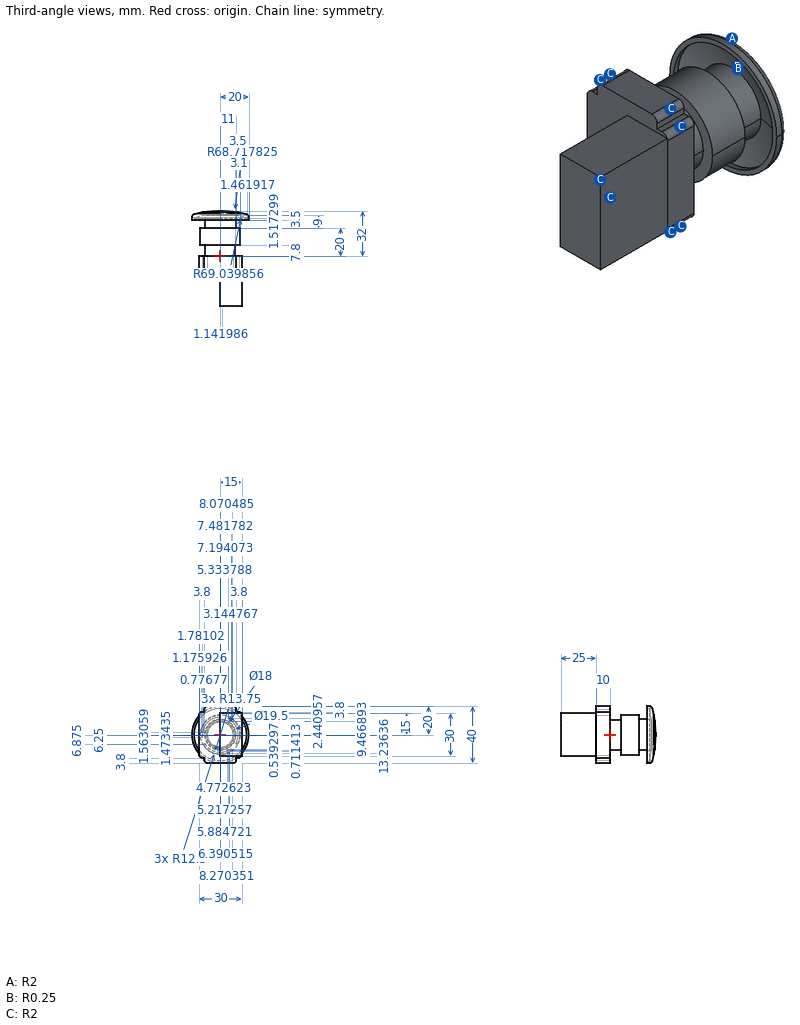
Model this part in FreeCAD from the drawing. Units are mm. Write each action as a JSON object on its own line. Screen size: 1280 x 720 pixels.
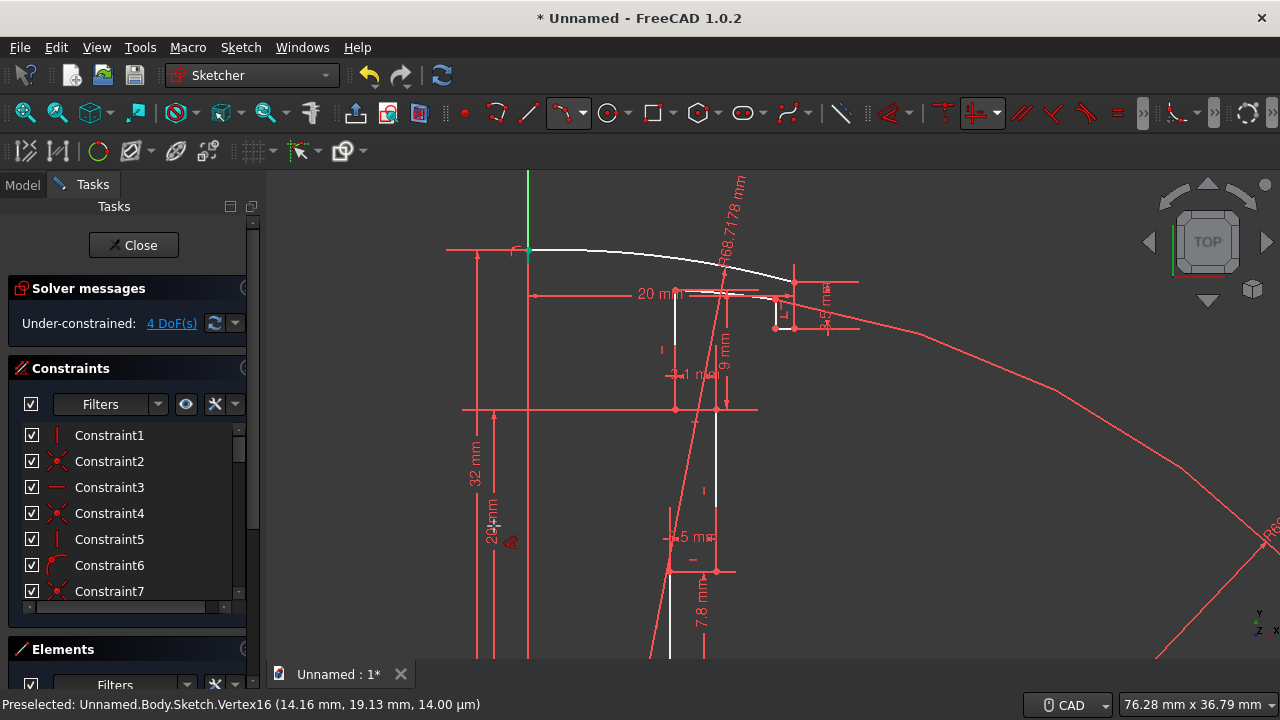
{"action": "left_click", "coordinate": [675, 410]}
{"action": "left_click", "coordinate": [602, 376]}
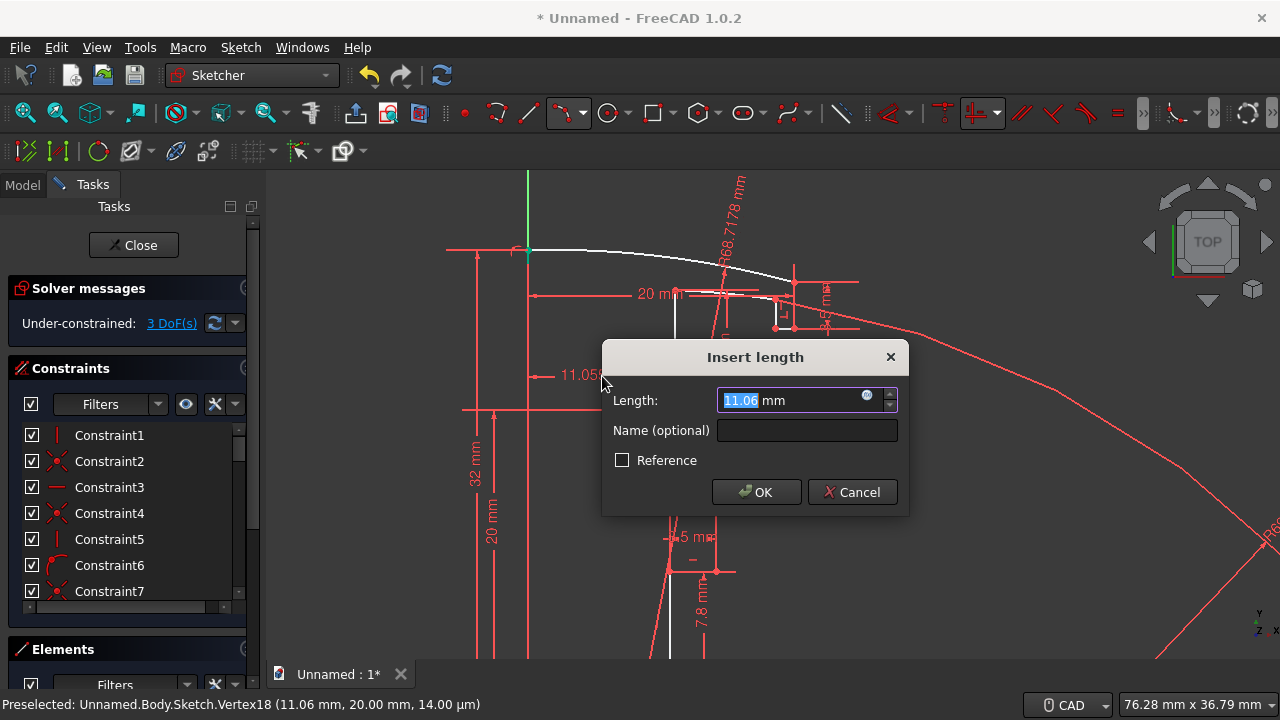
{"action": "type", "text": "11"}
{"action": "key", "text": "Return"}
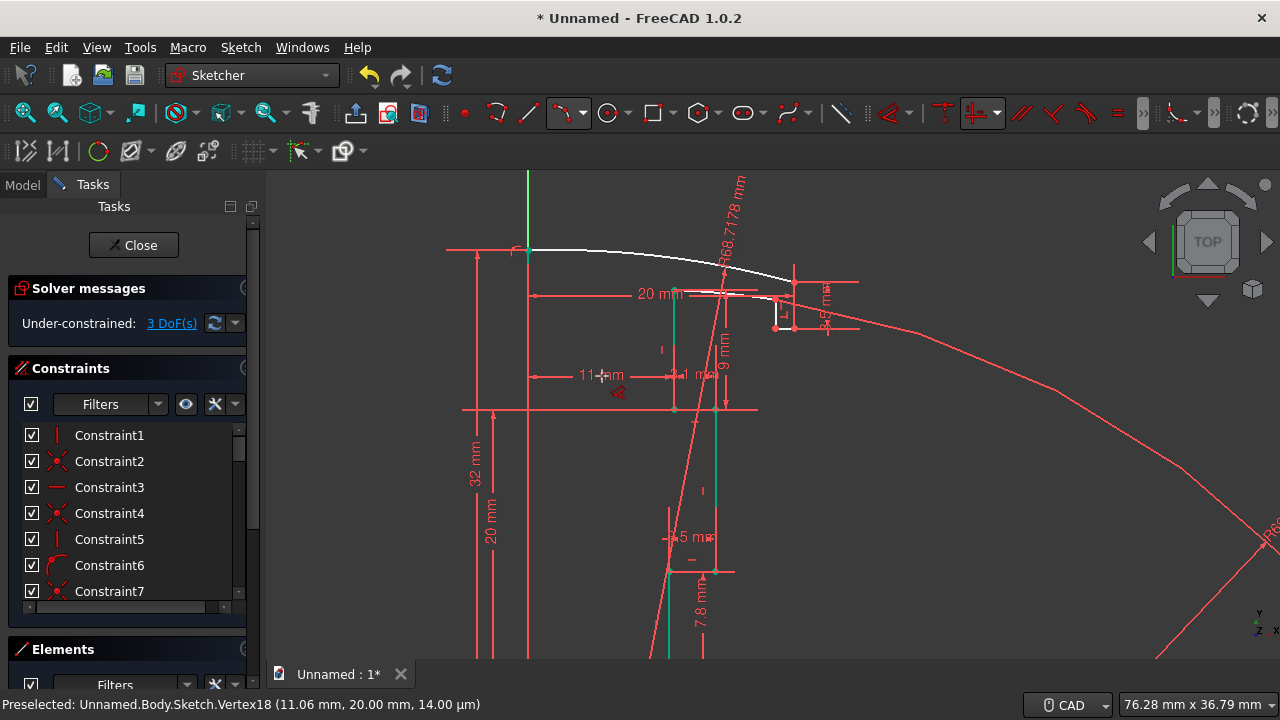
{"action": "scroll", "coordinate": [776, 311], "scroll_direction": "up", "scroll_amount": 4}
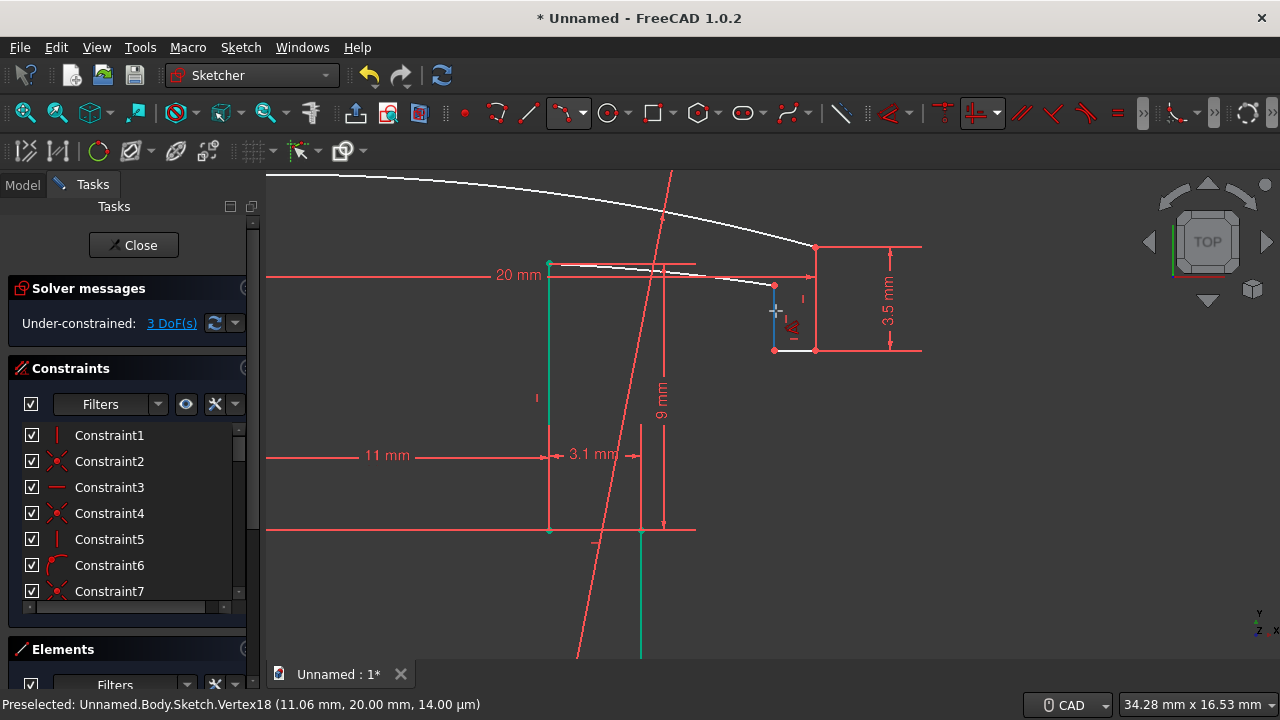
{"action": "left_click", "coordinate": [774, 312]}
{"action": "left_click", "coordinate": [740, 318]}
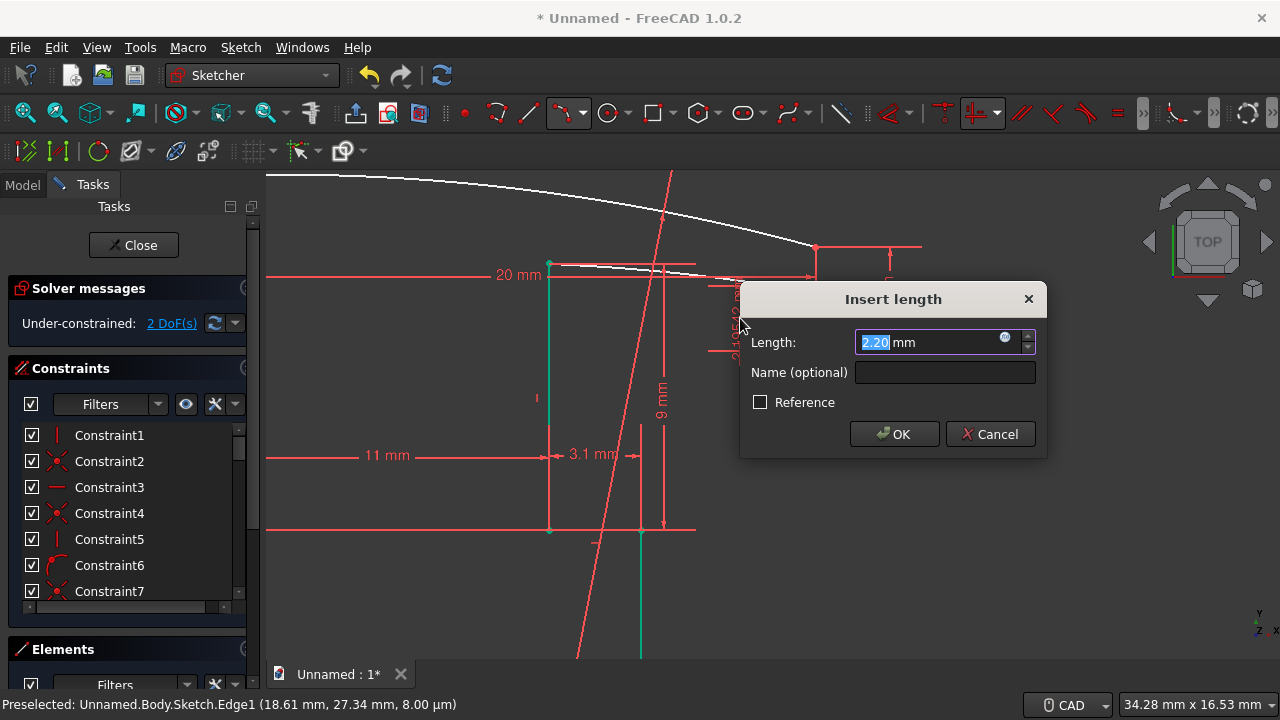
{"action": "type", "text": "1.517299"}
{"action": "key", "text": "Return"}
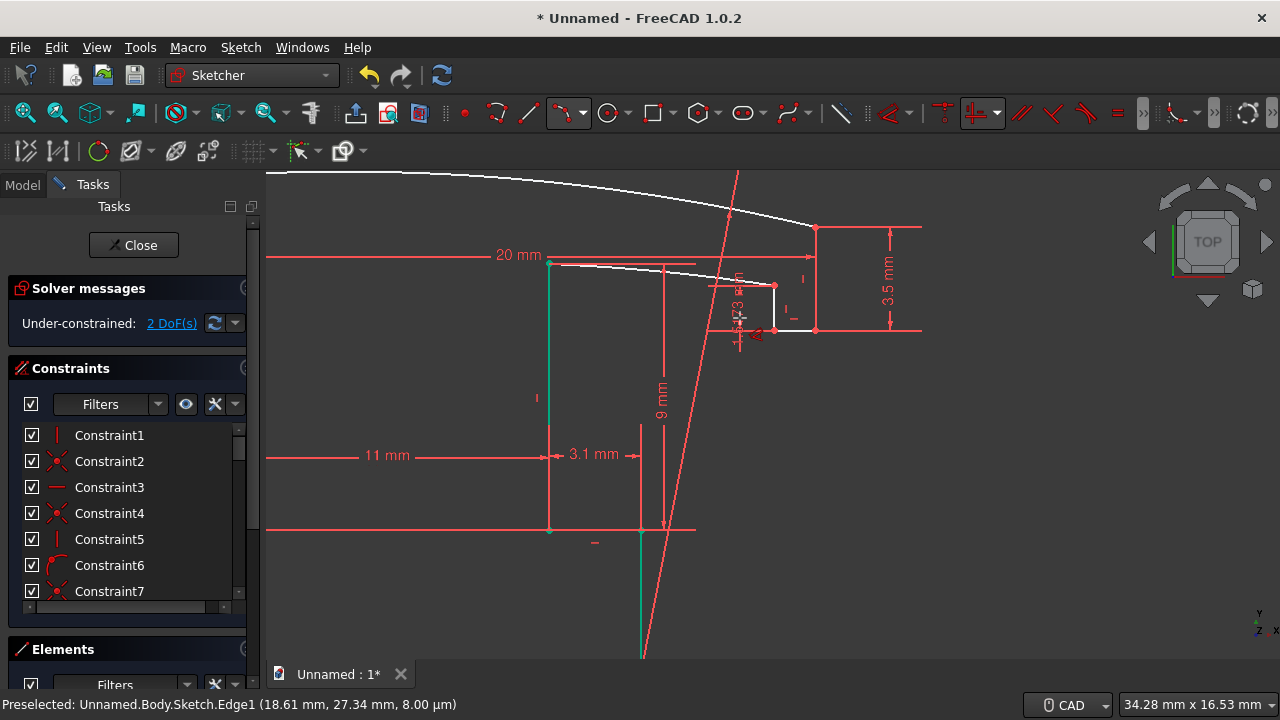
{"action": "left_click", "coordinate": [787, 331]}
{"action": "left_click", "coordinate": [795, 297]}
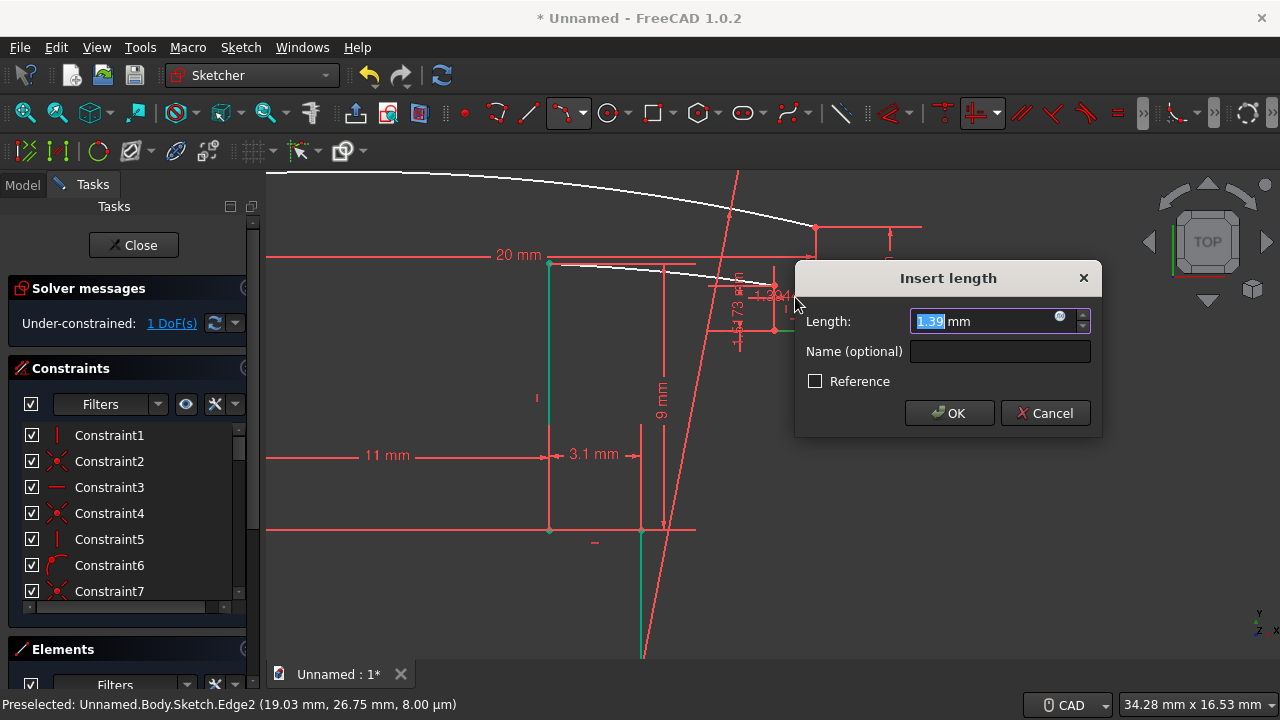
{"action": "type", "text": "1.461917"}
{"action": "key", "text": "Return"}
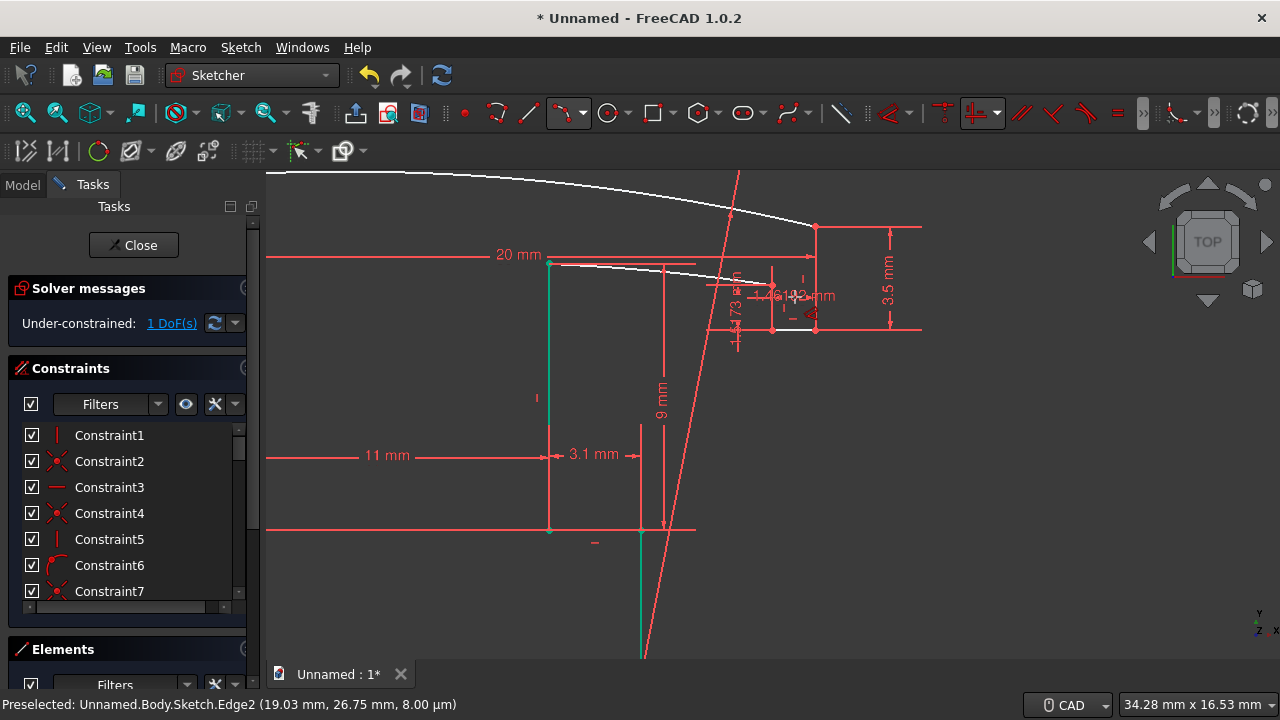
{"action": "scroll", "coordinate": [784, 314], "scroll_direction": "down", "scroll_amount": 6}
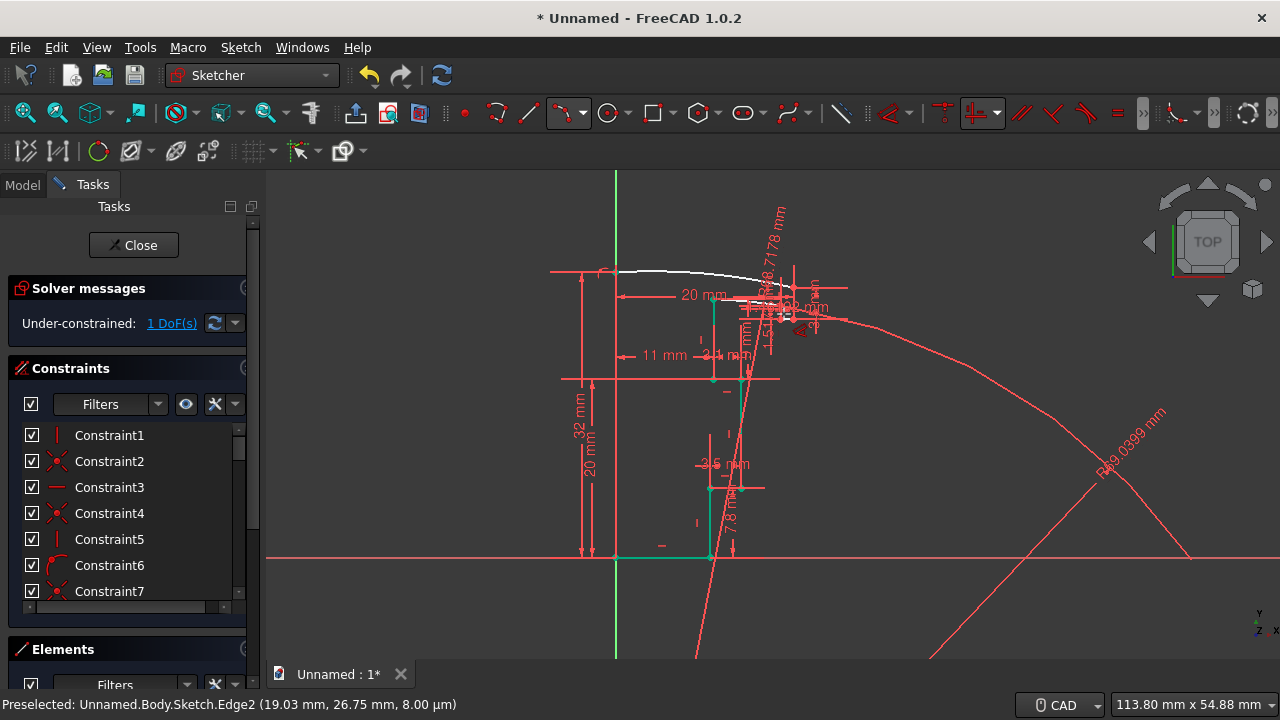
{"action": "scroll", "coordinate": [704, 216], "scroll_direction": "down", "scroll_amount": 3}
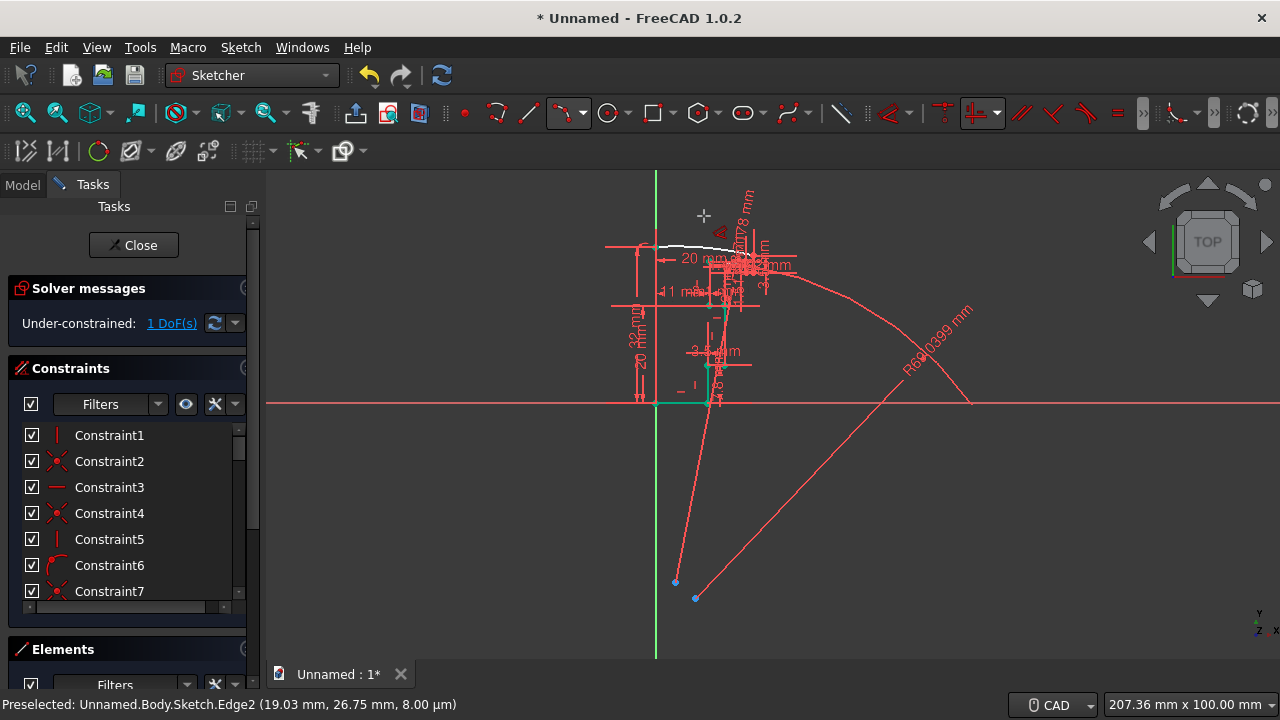
{"action": "scroll", "coordinate": [676, 582], "scroll_direction": "up", "scroll_amount": 10}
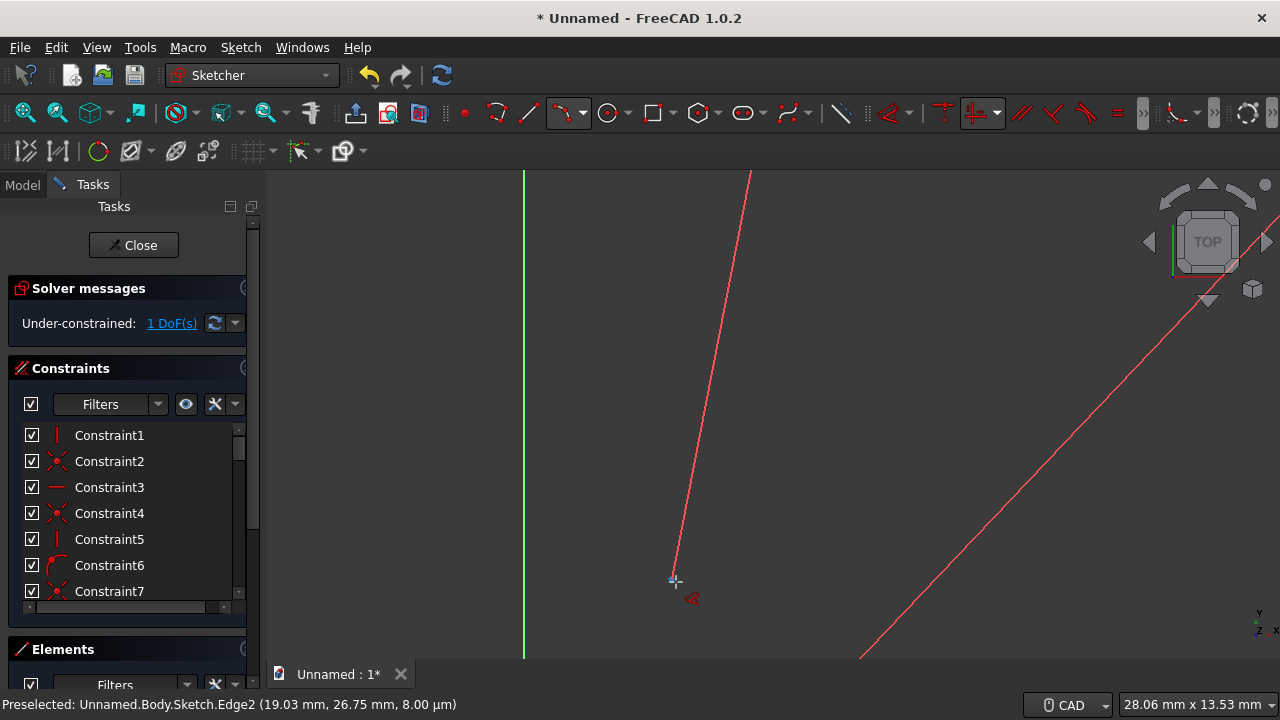
{"action": "left_click", "coordinate": [672, 580]}
{"action": "left_click", "coordinate": [598, 614]}